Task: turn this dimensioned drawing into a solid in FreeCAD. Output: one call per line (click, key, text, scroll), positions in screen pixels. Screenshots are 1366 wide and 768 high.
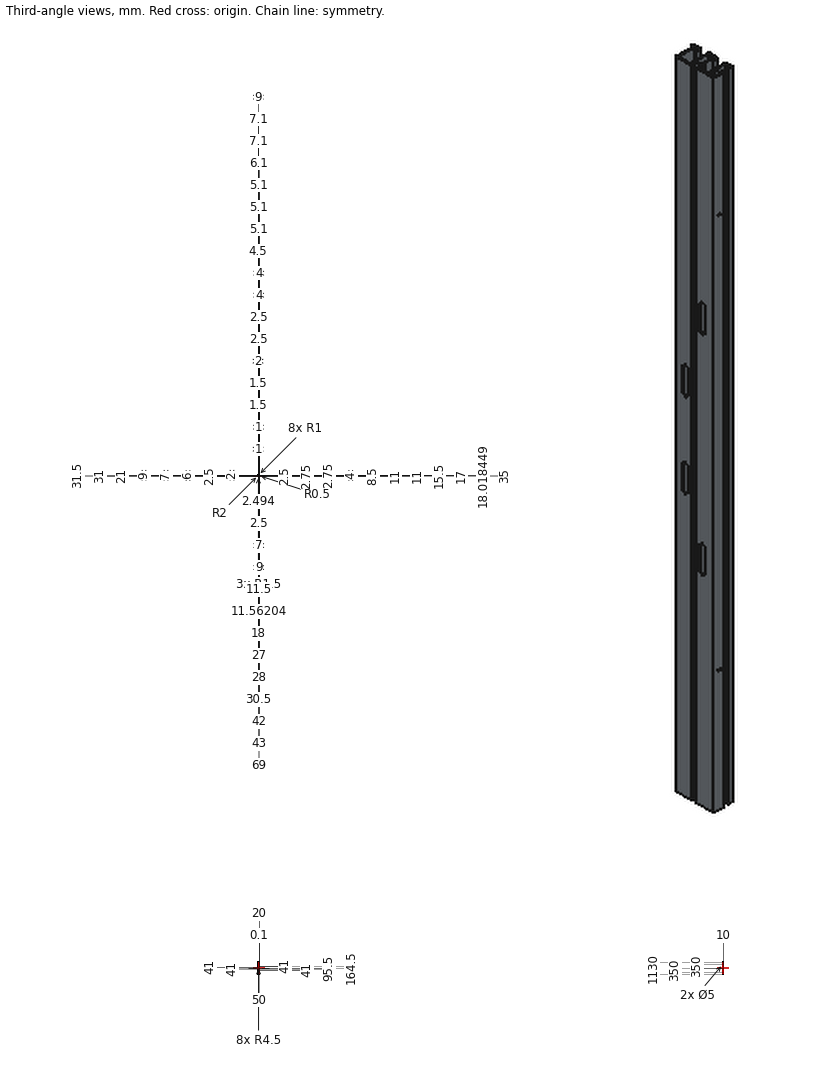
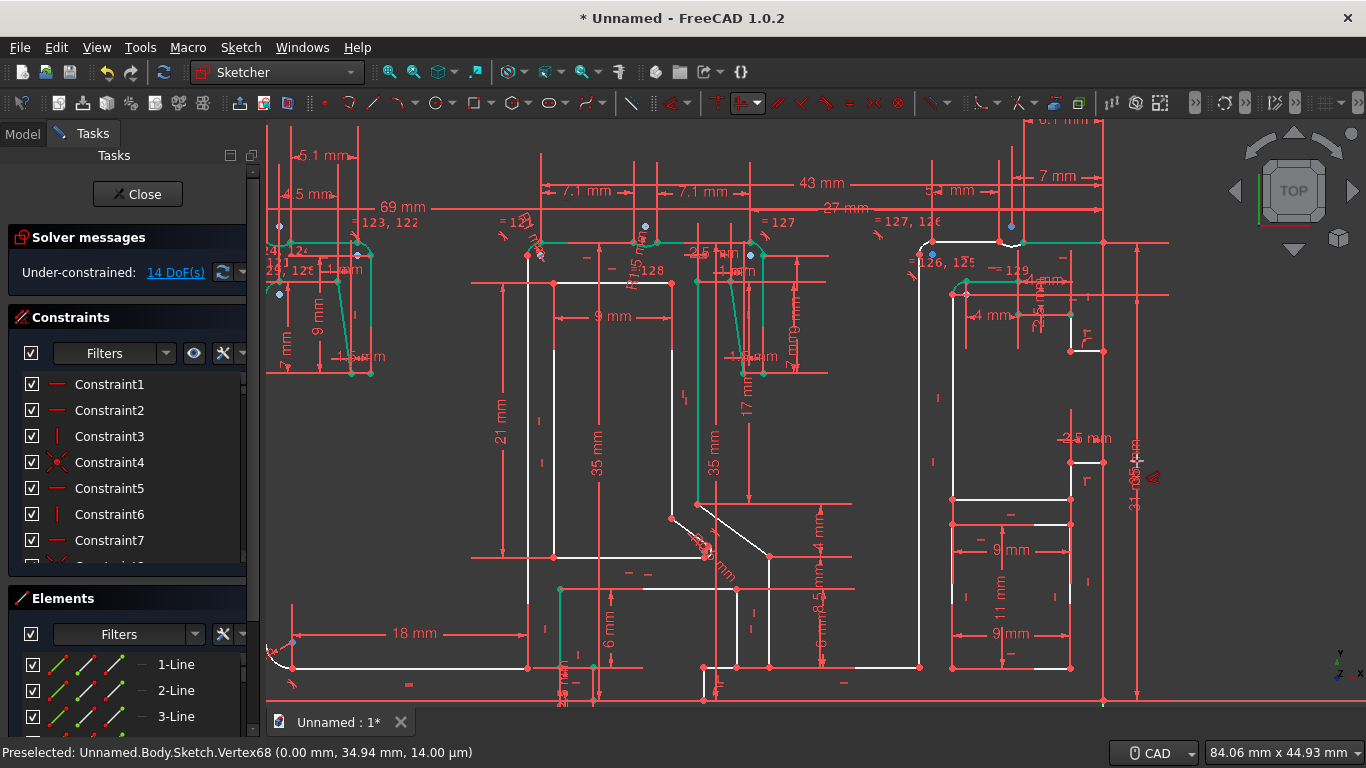
click(999, 242)
click(1137, 360)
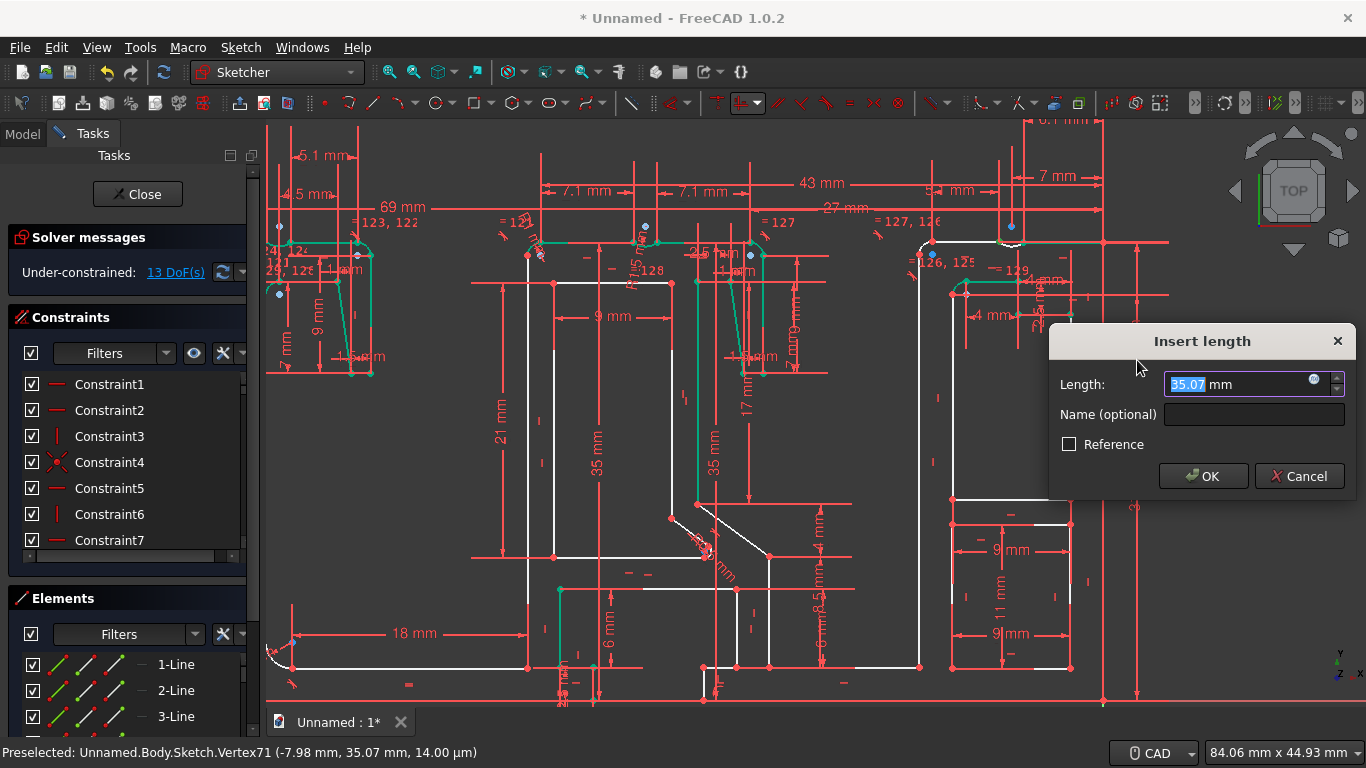
text(35)
key(Return)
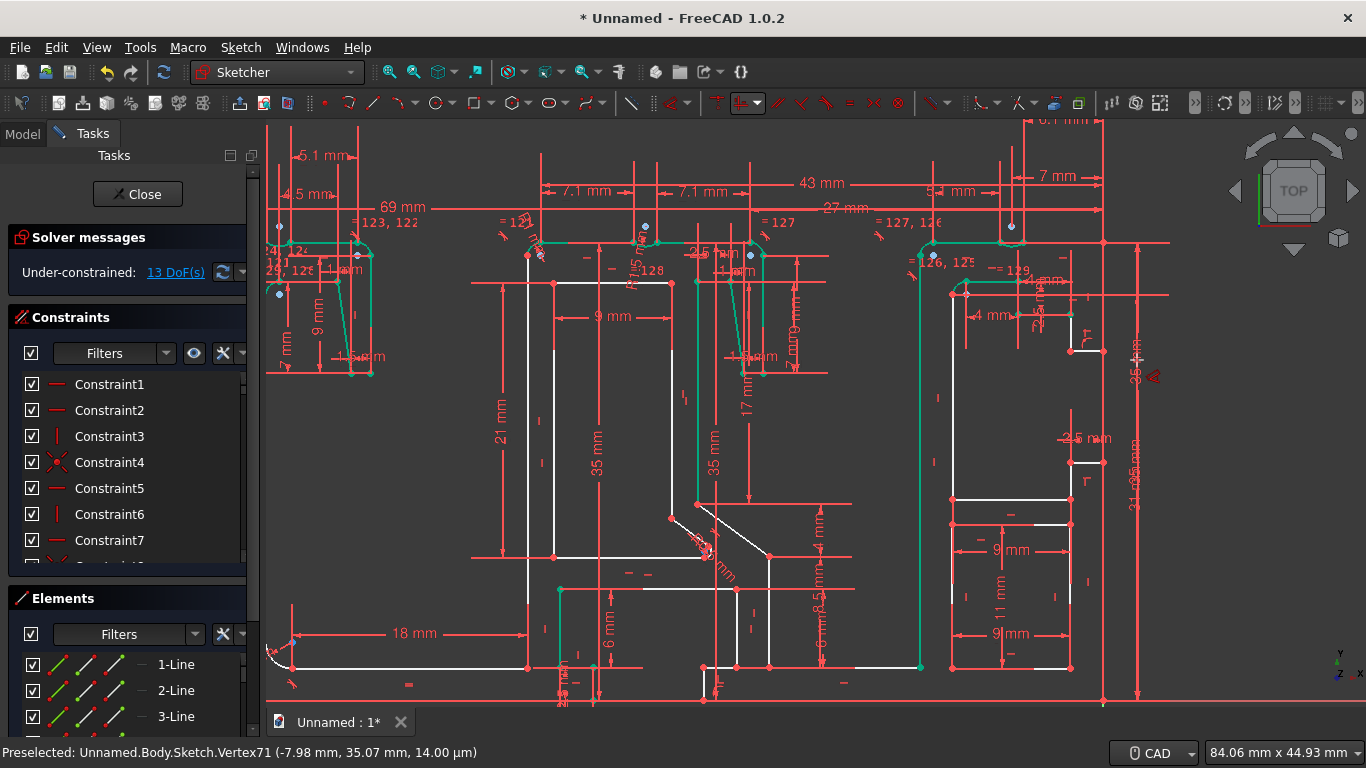
scroll(705, 558, up, 4)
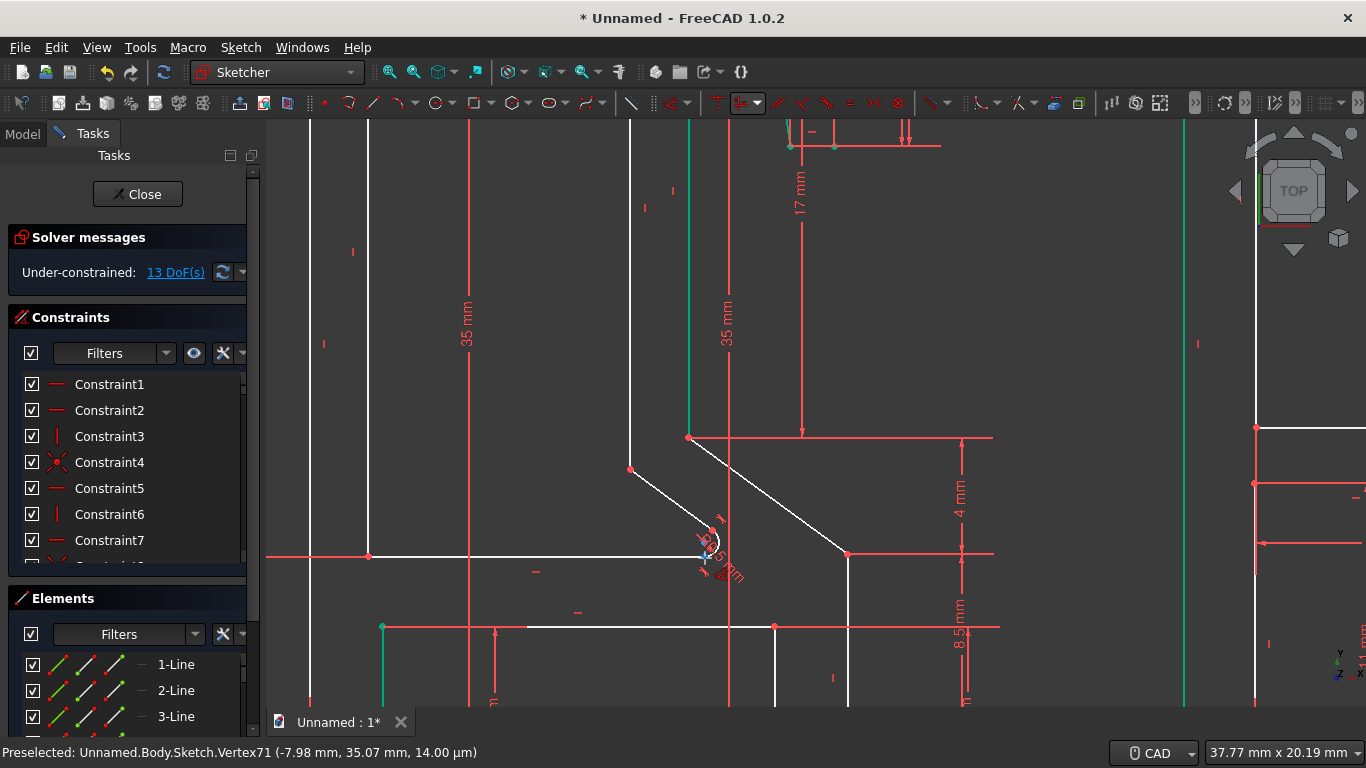
click(704, 557)
click(670, 590)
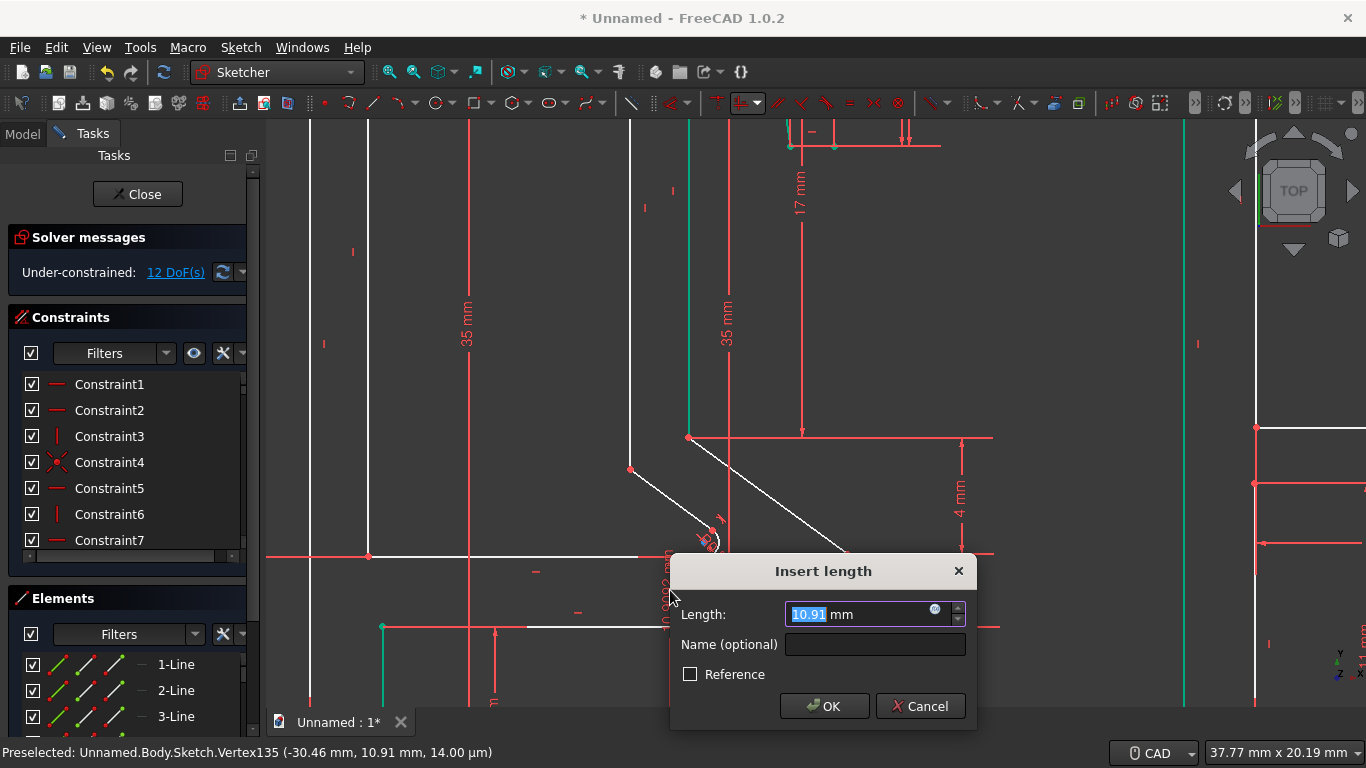
text(11)
key(Return)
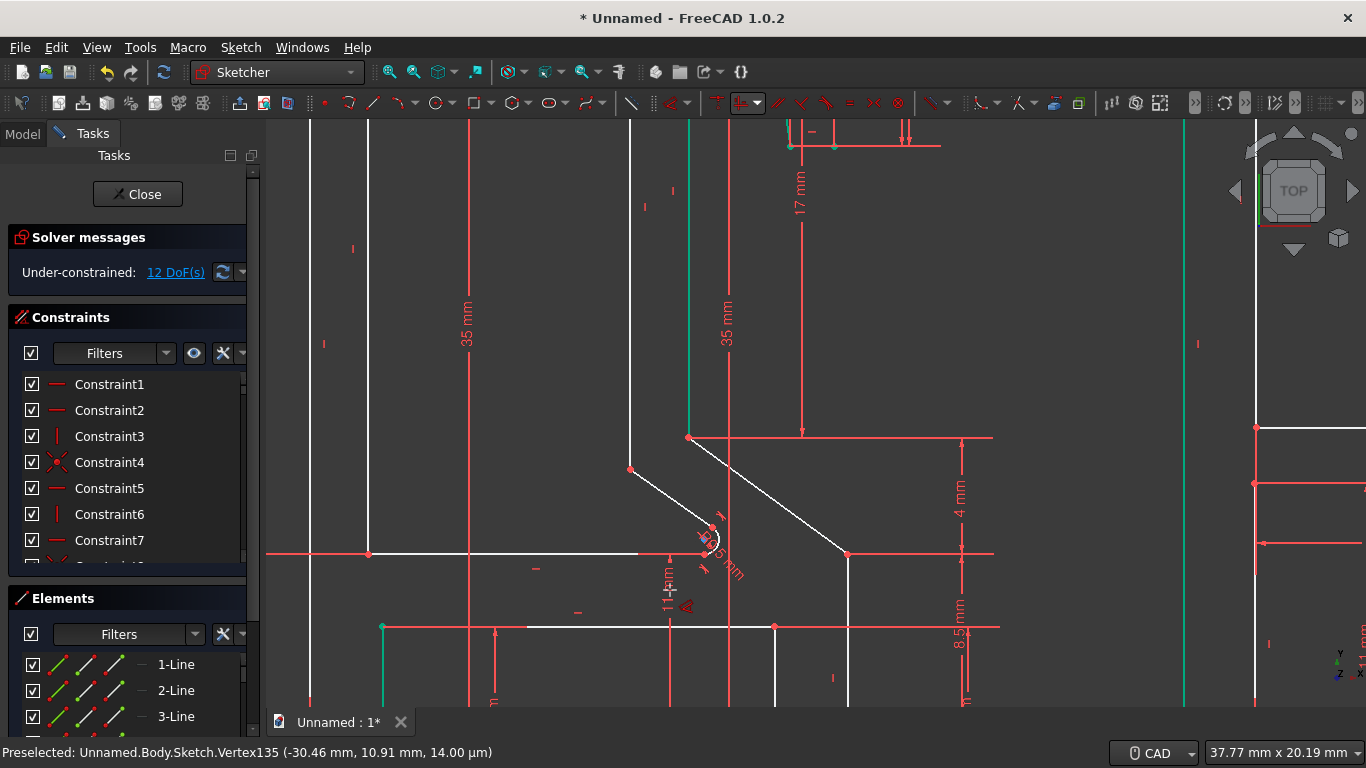
click(368, 554)
click(593, 520)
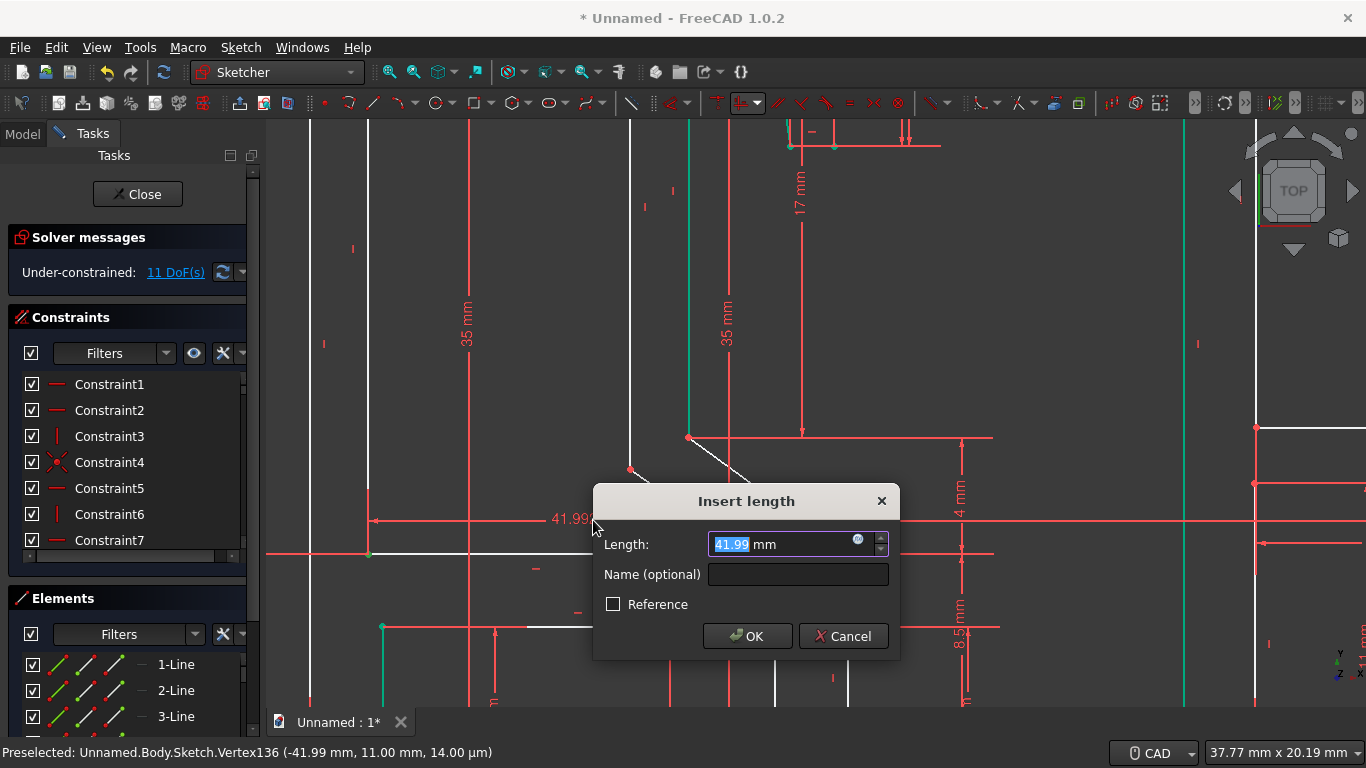
text(42)
key(Return)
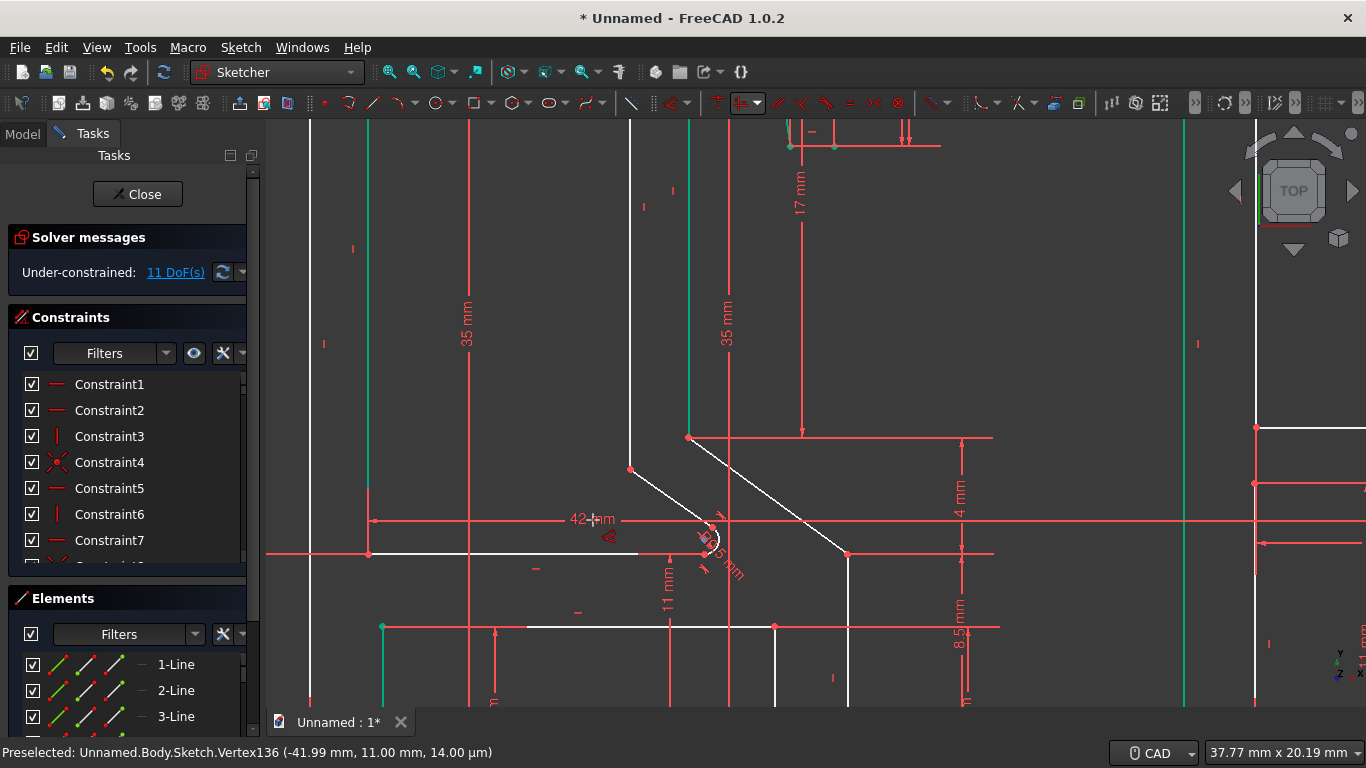
click(310, 160)
click(344, 413)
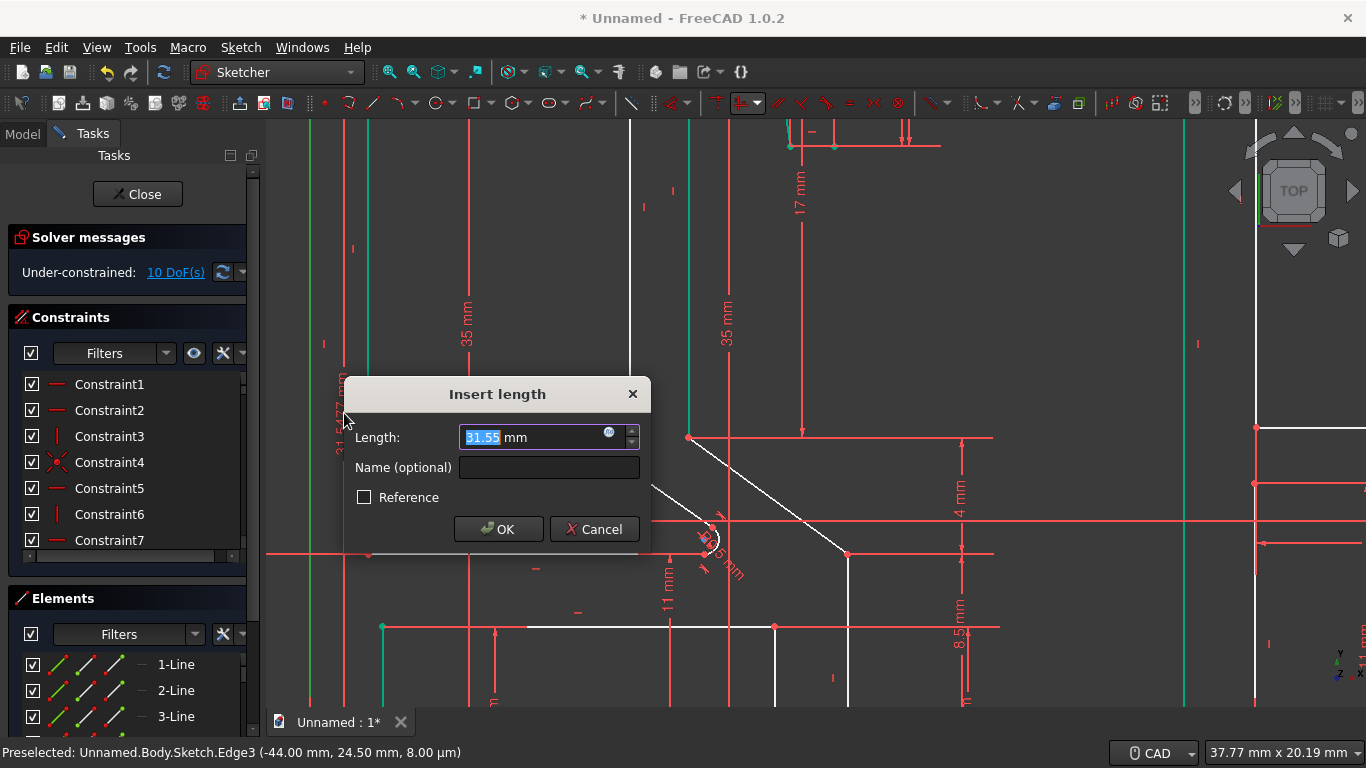
text(31.5)
key(Return)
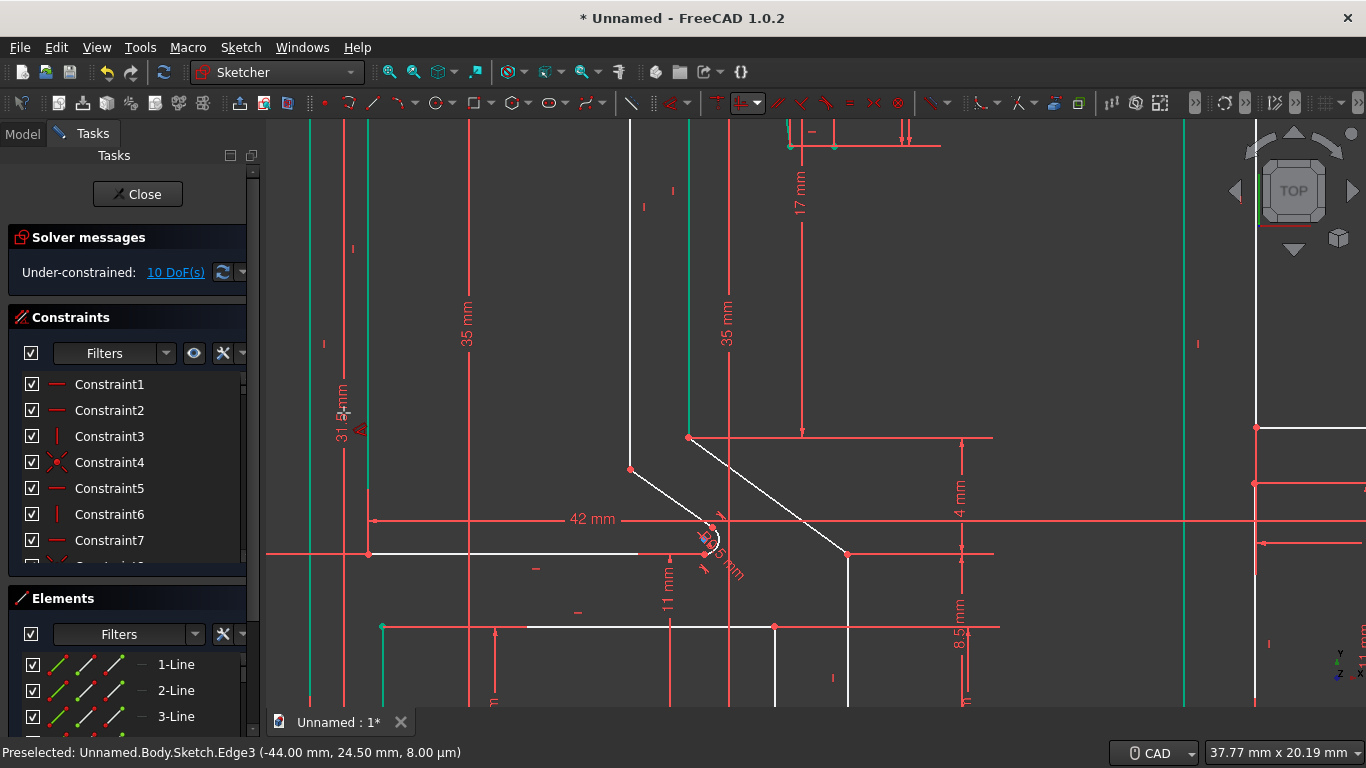
scroll(823, 434, down, 6)